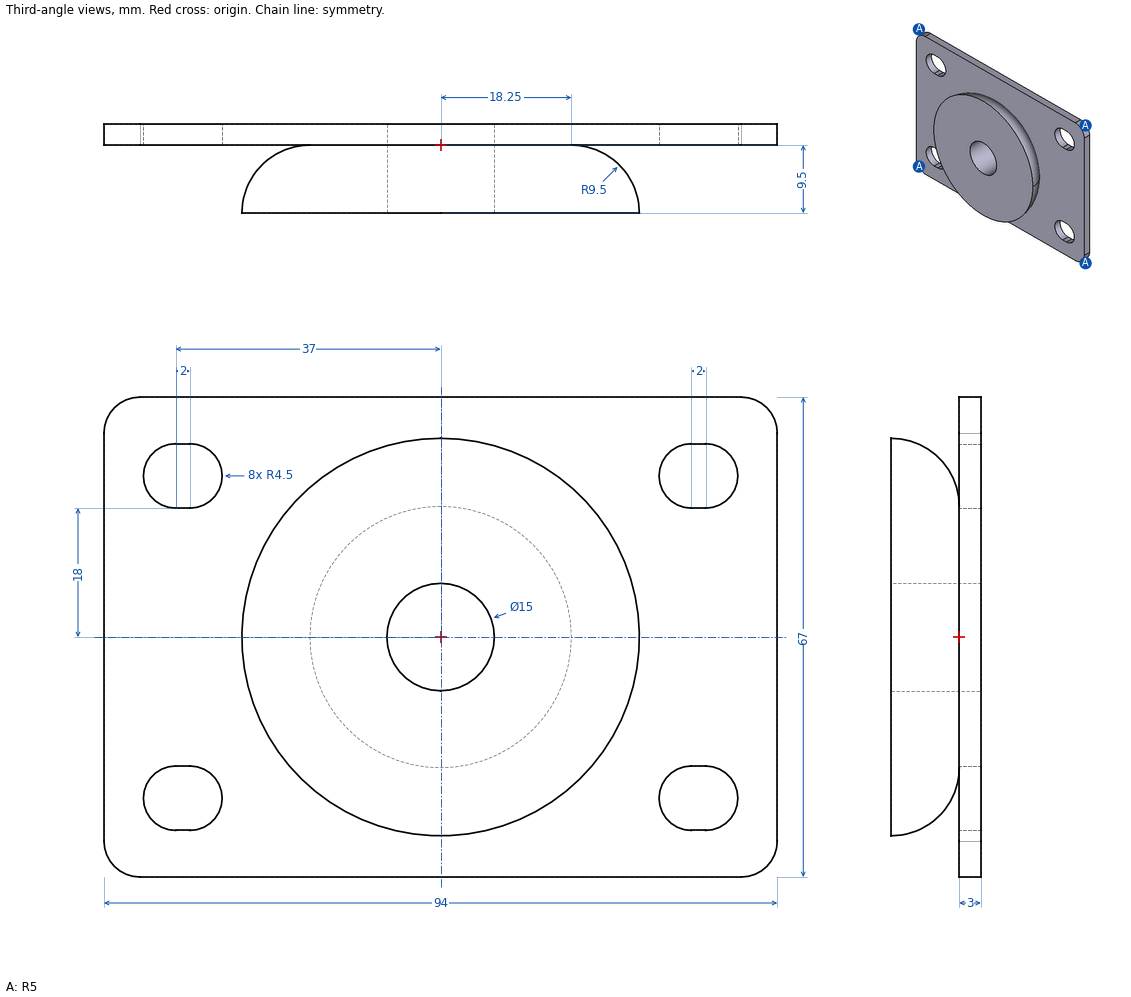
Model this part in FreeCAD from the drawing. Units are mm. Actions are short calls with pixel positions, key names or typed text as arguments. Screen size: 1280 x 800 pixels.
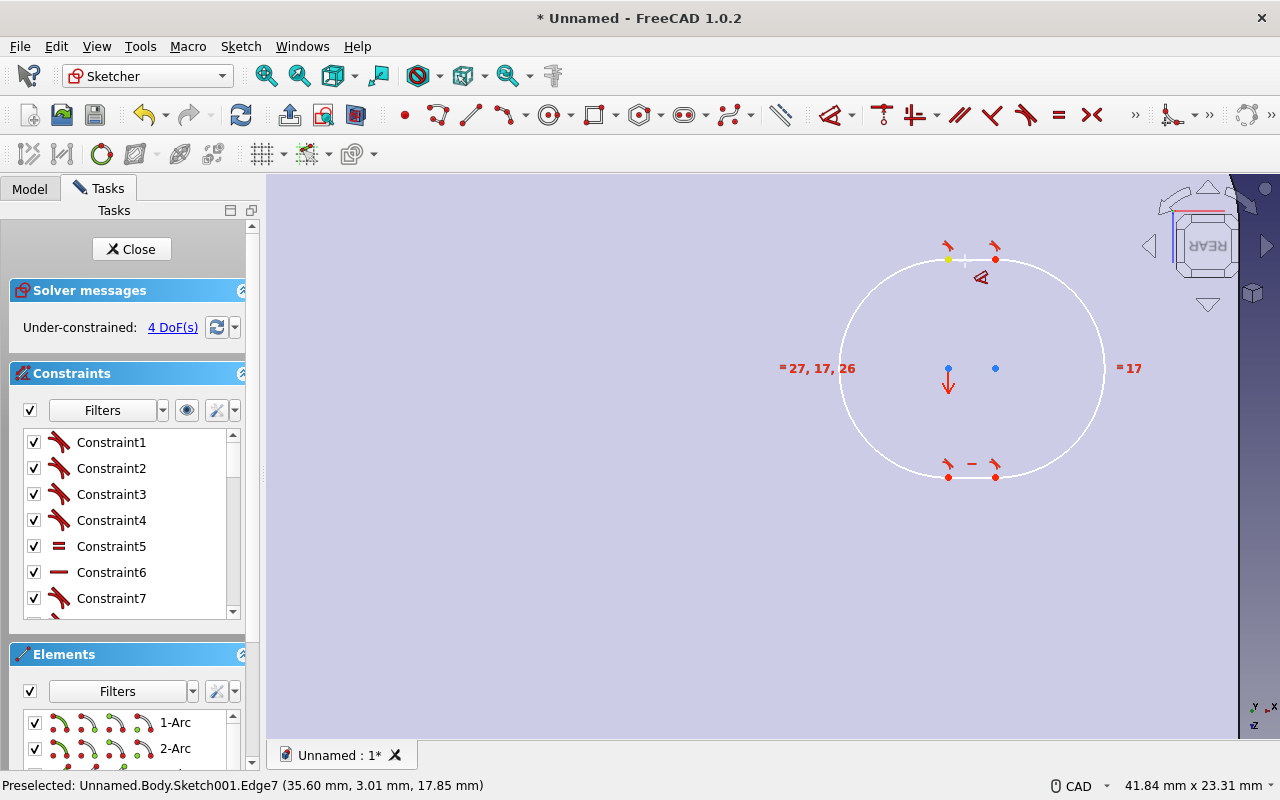
click(963, 260)
click(972, 226)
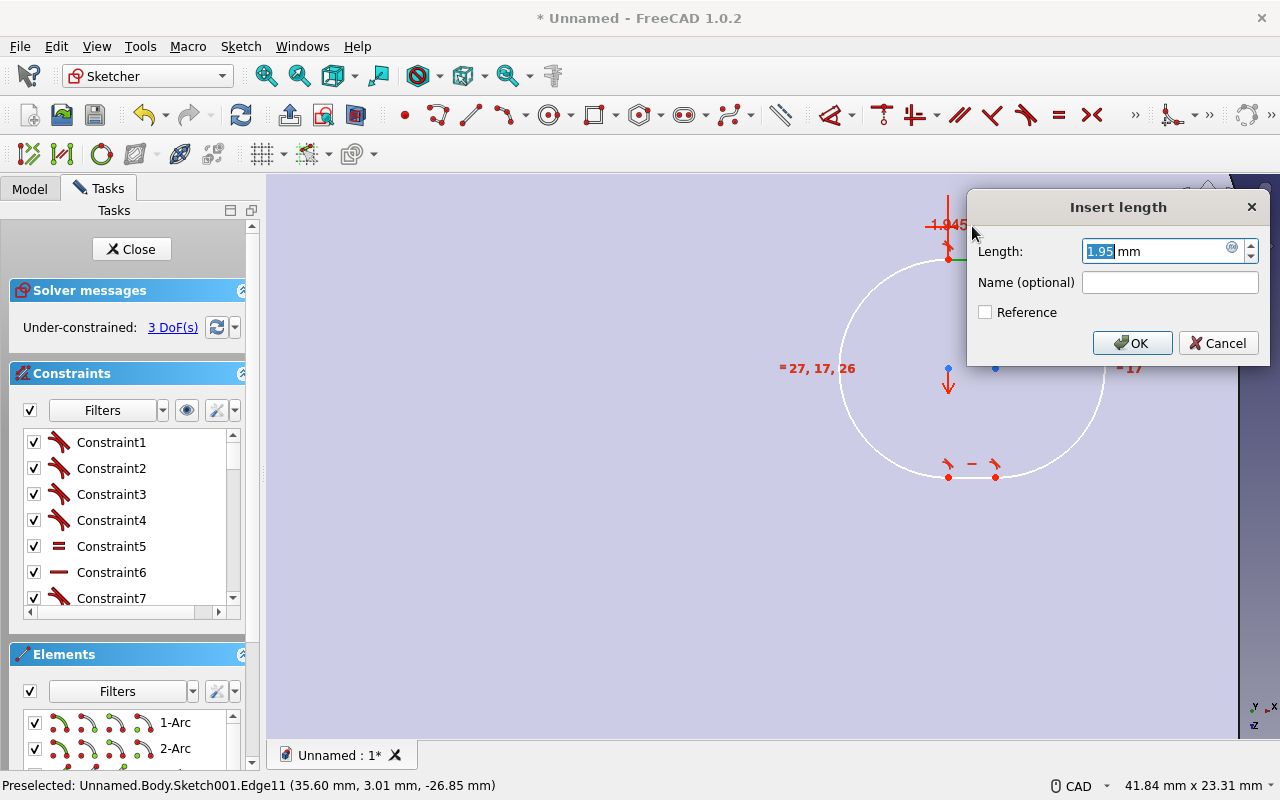
text(2)
key(Return)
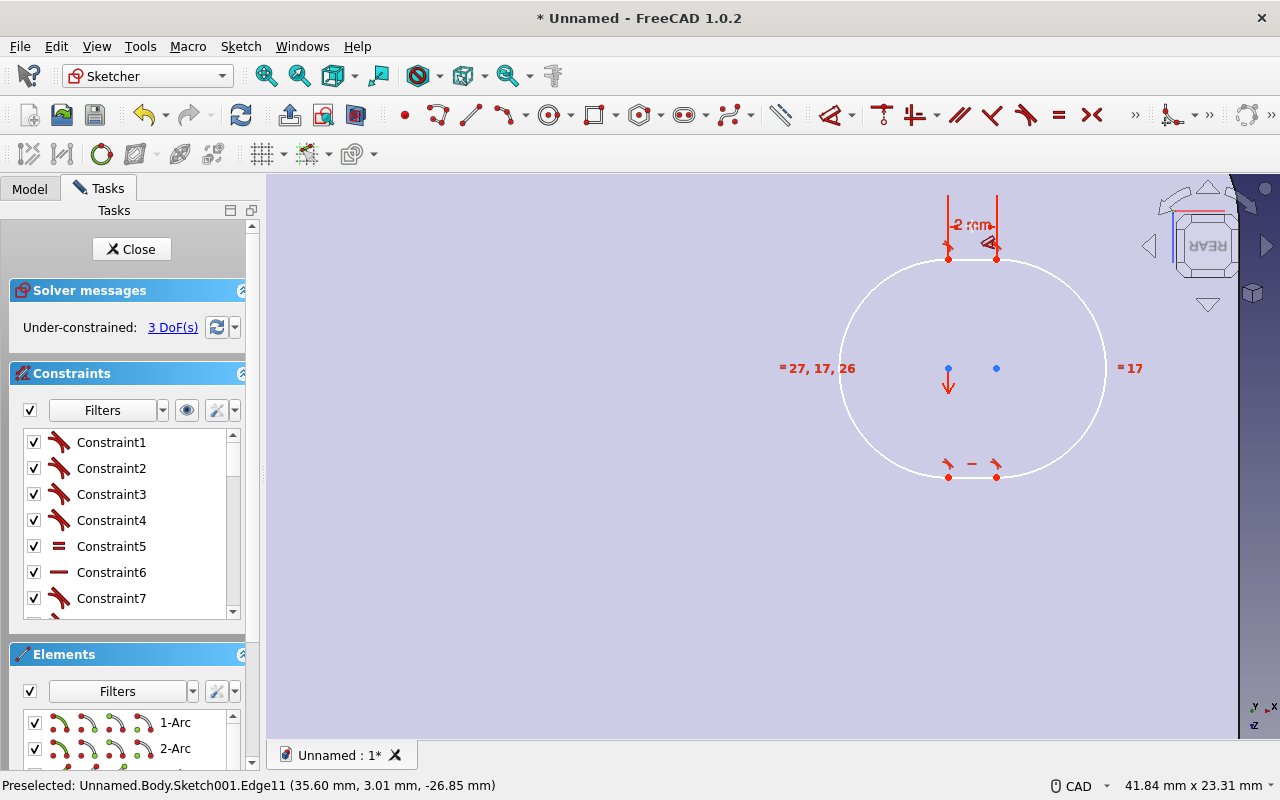
scroll(965, 261, down, 6)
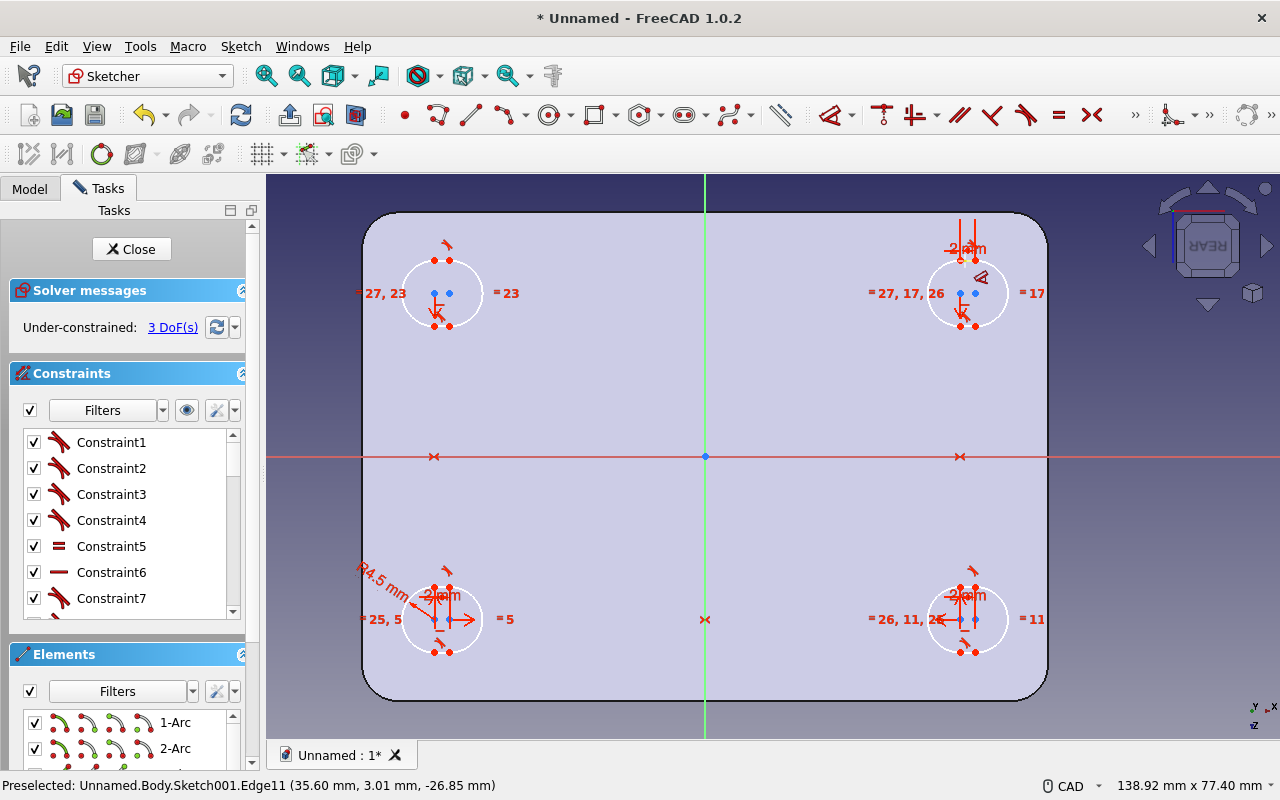
scroll(439, 261, up, 6)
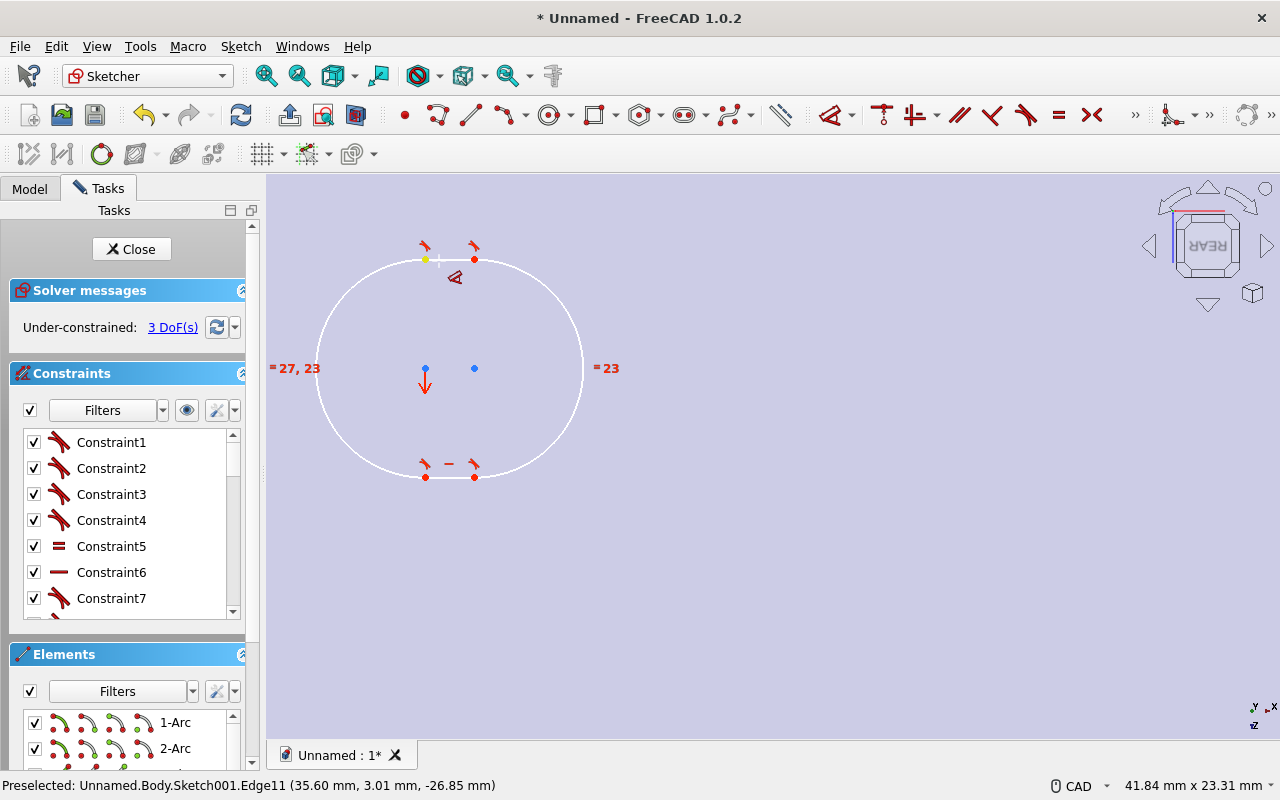
click(440, 260)
click(450, 226)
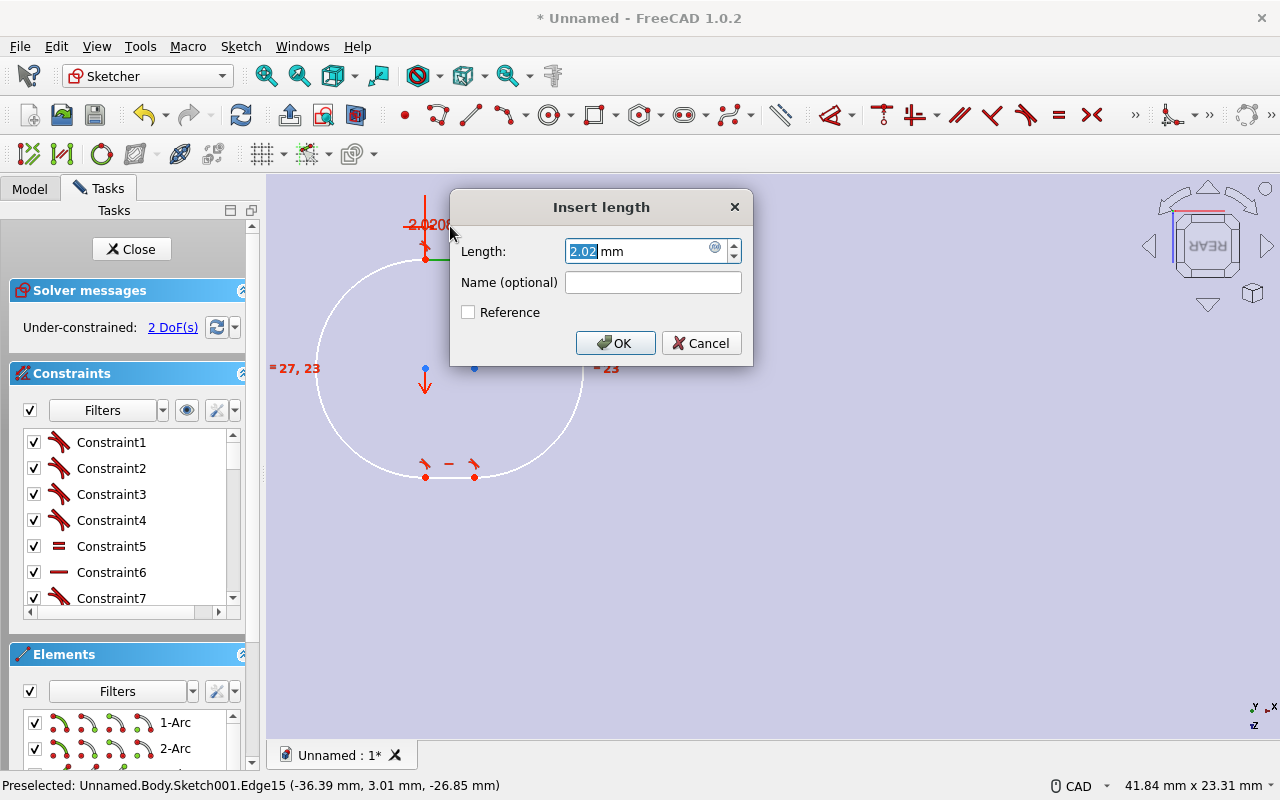
text(2)
key(Return)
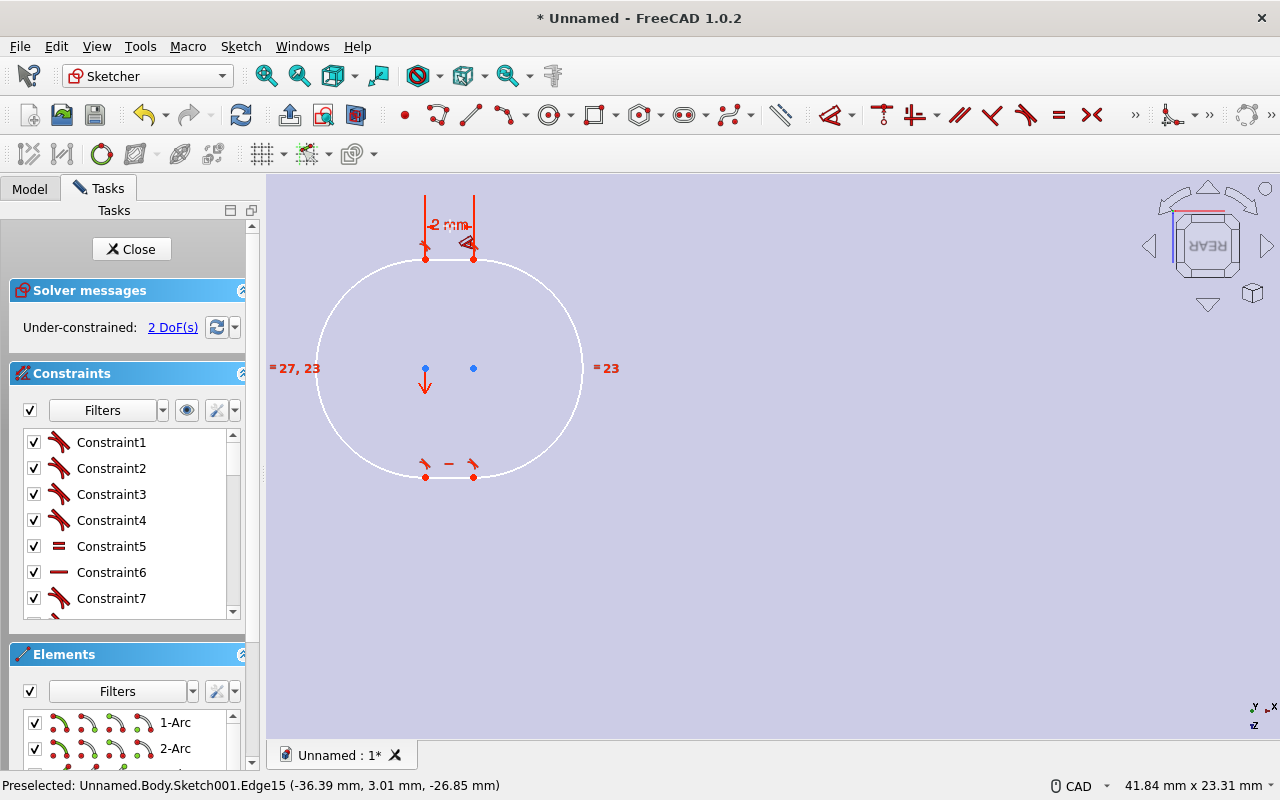
scroll(438, 261, down, 6)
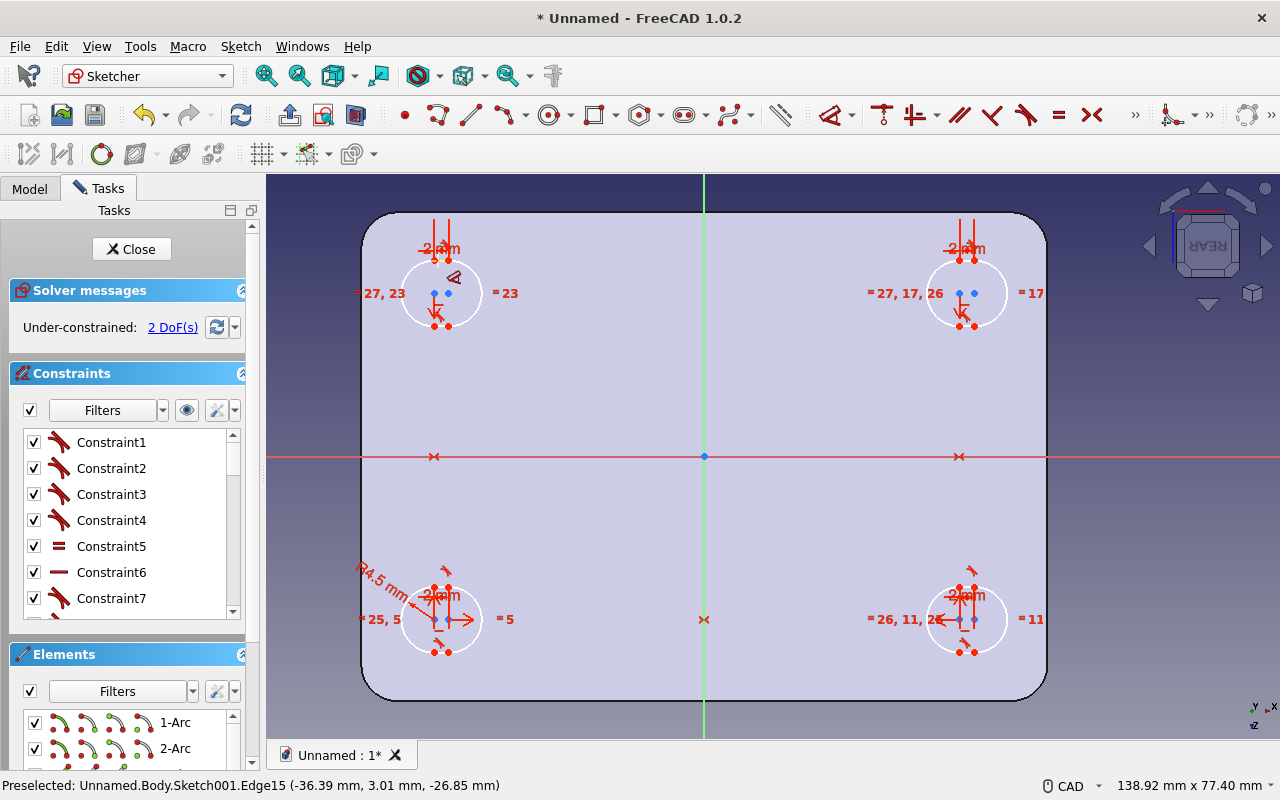
click(434, 587)
click(569, 621)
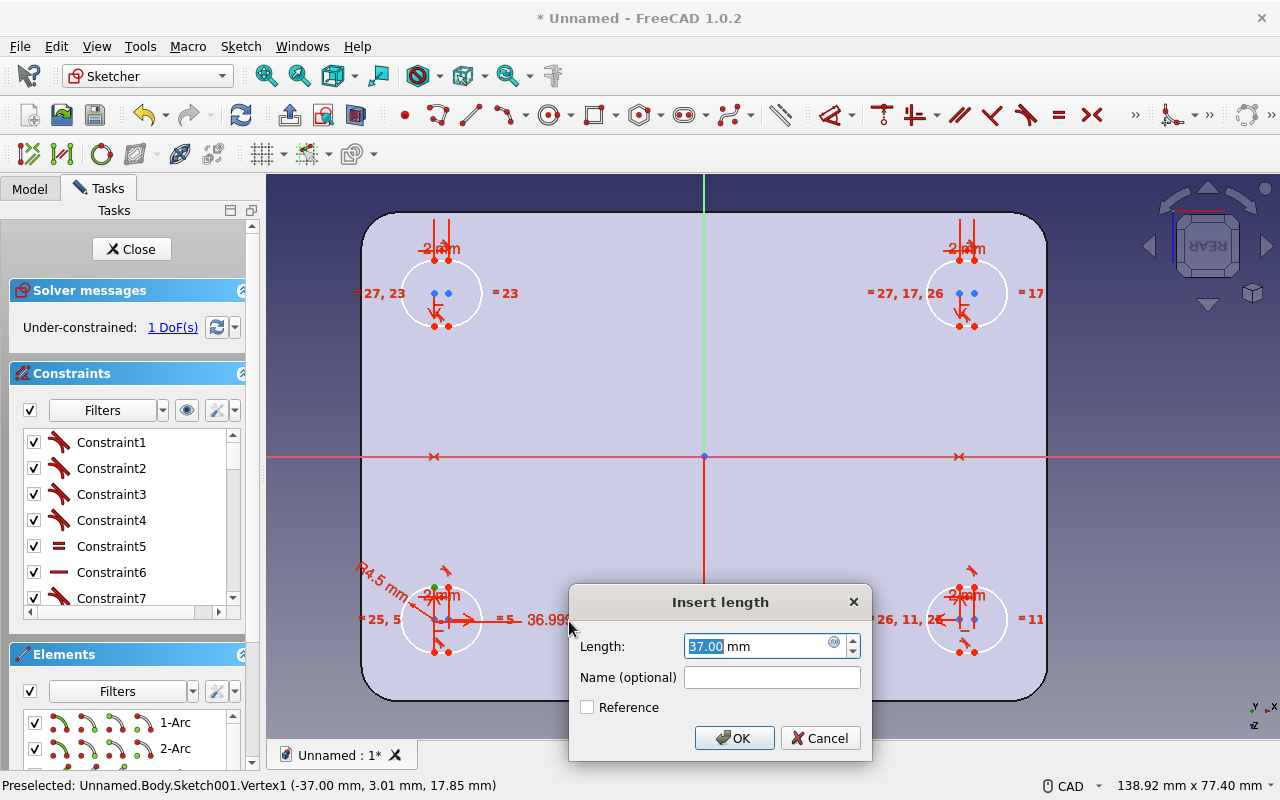
text(37)
key(Return)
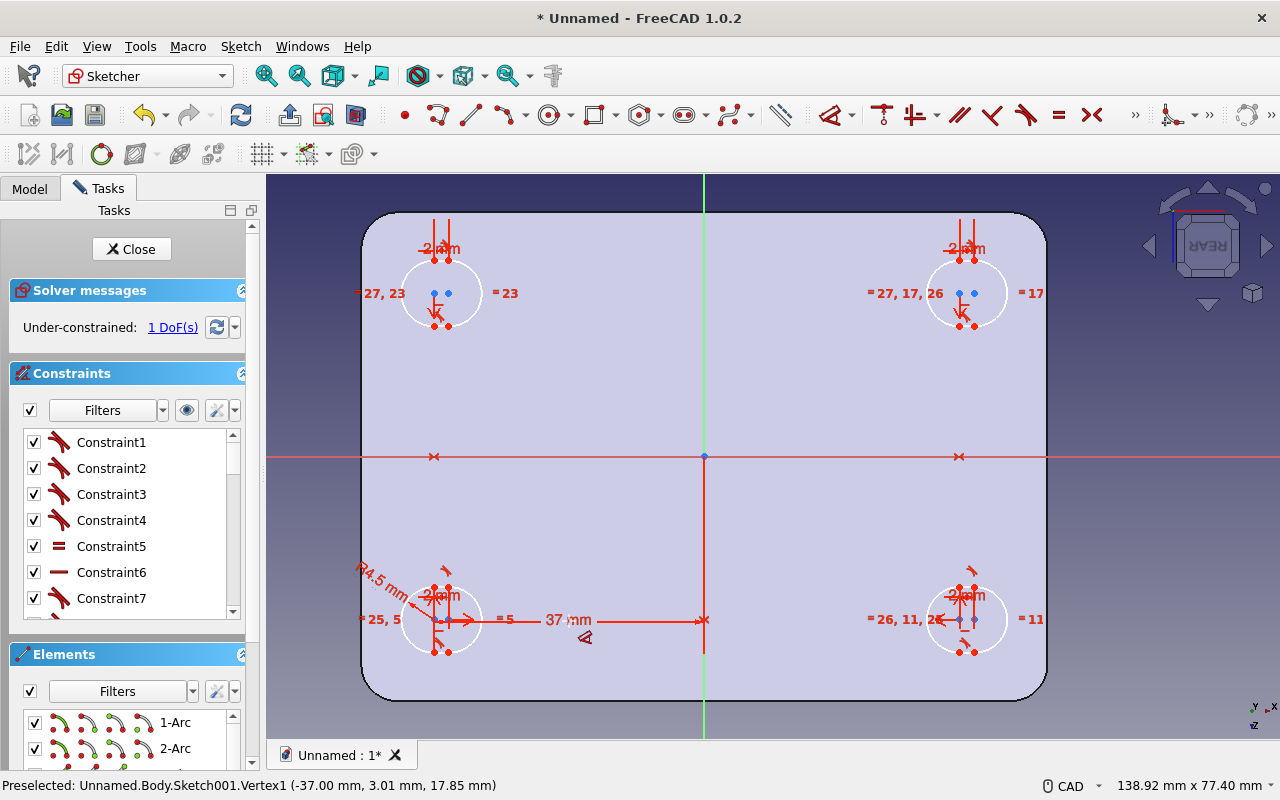
click(434, 587)
click(400, 522)